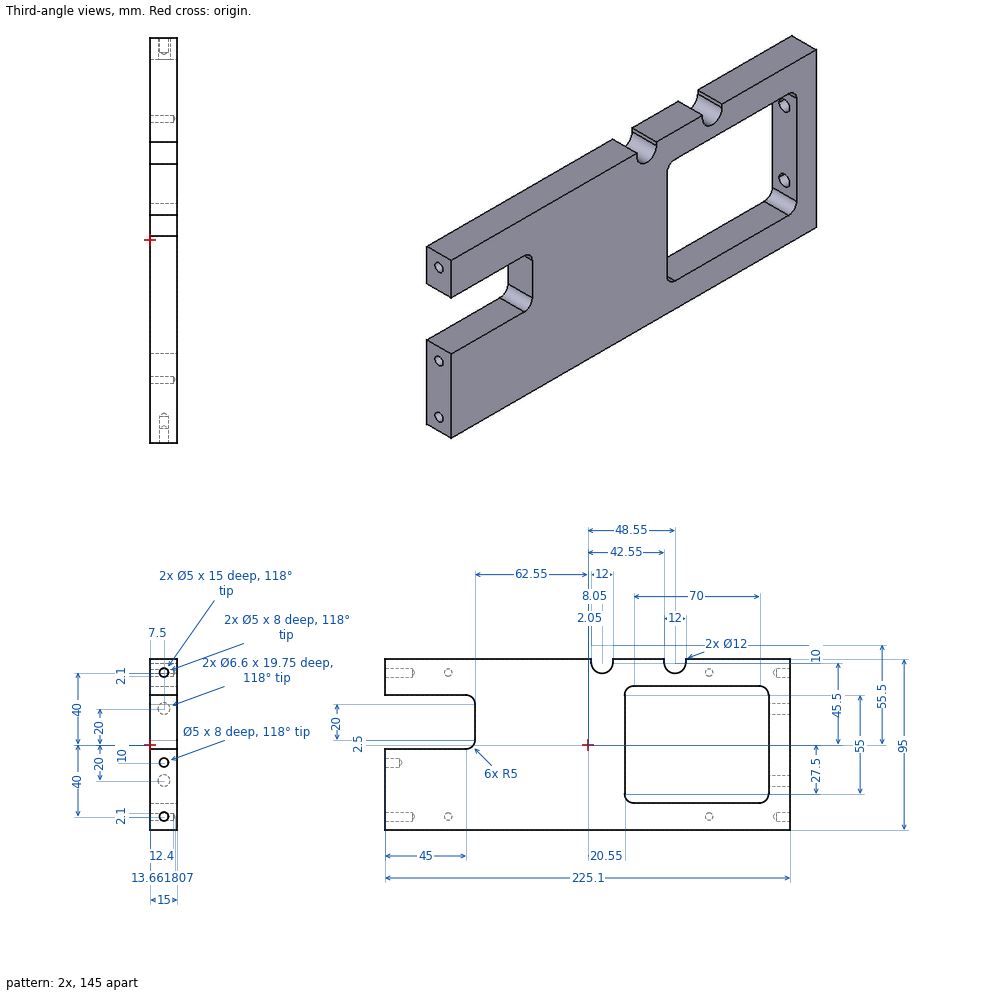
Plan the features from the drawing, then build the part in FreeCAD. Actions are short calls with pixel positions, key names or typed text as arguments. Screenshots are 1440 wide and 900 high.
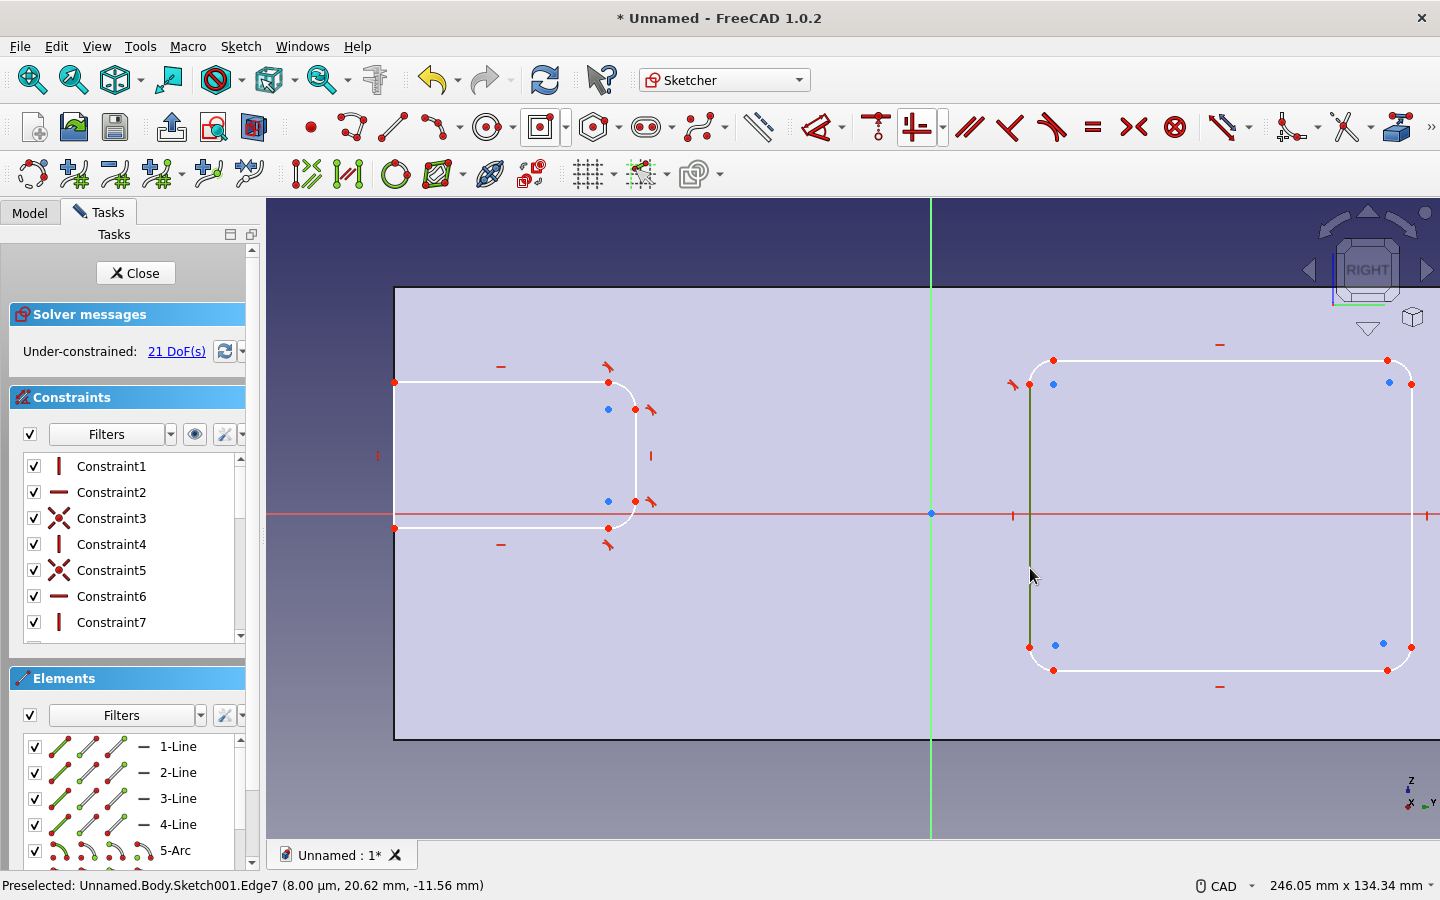
scroll(1033, 658, up, 2)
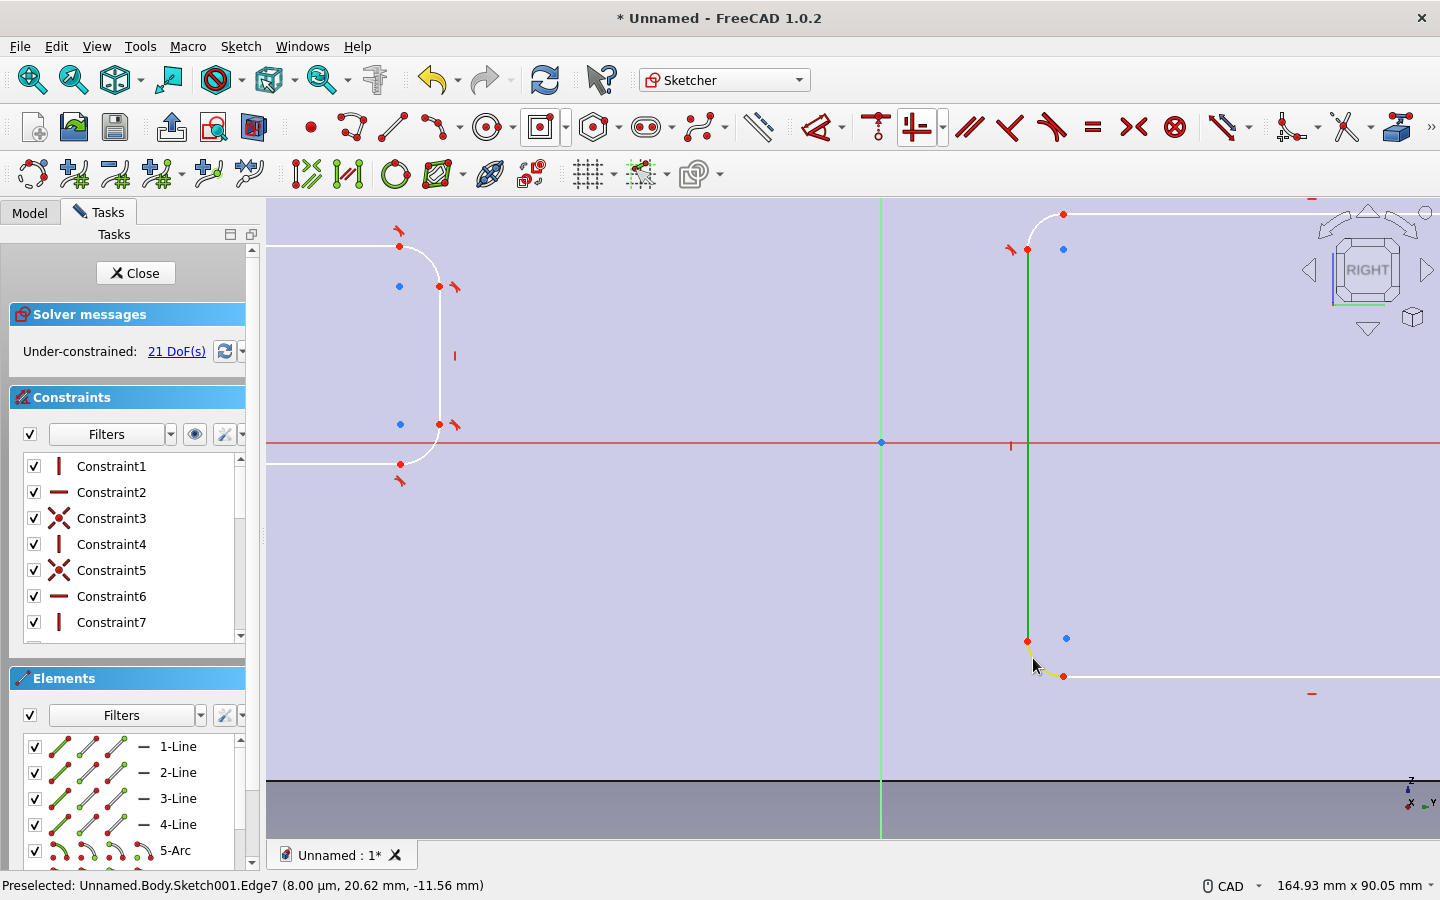
click(1032, 657)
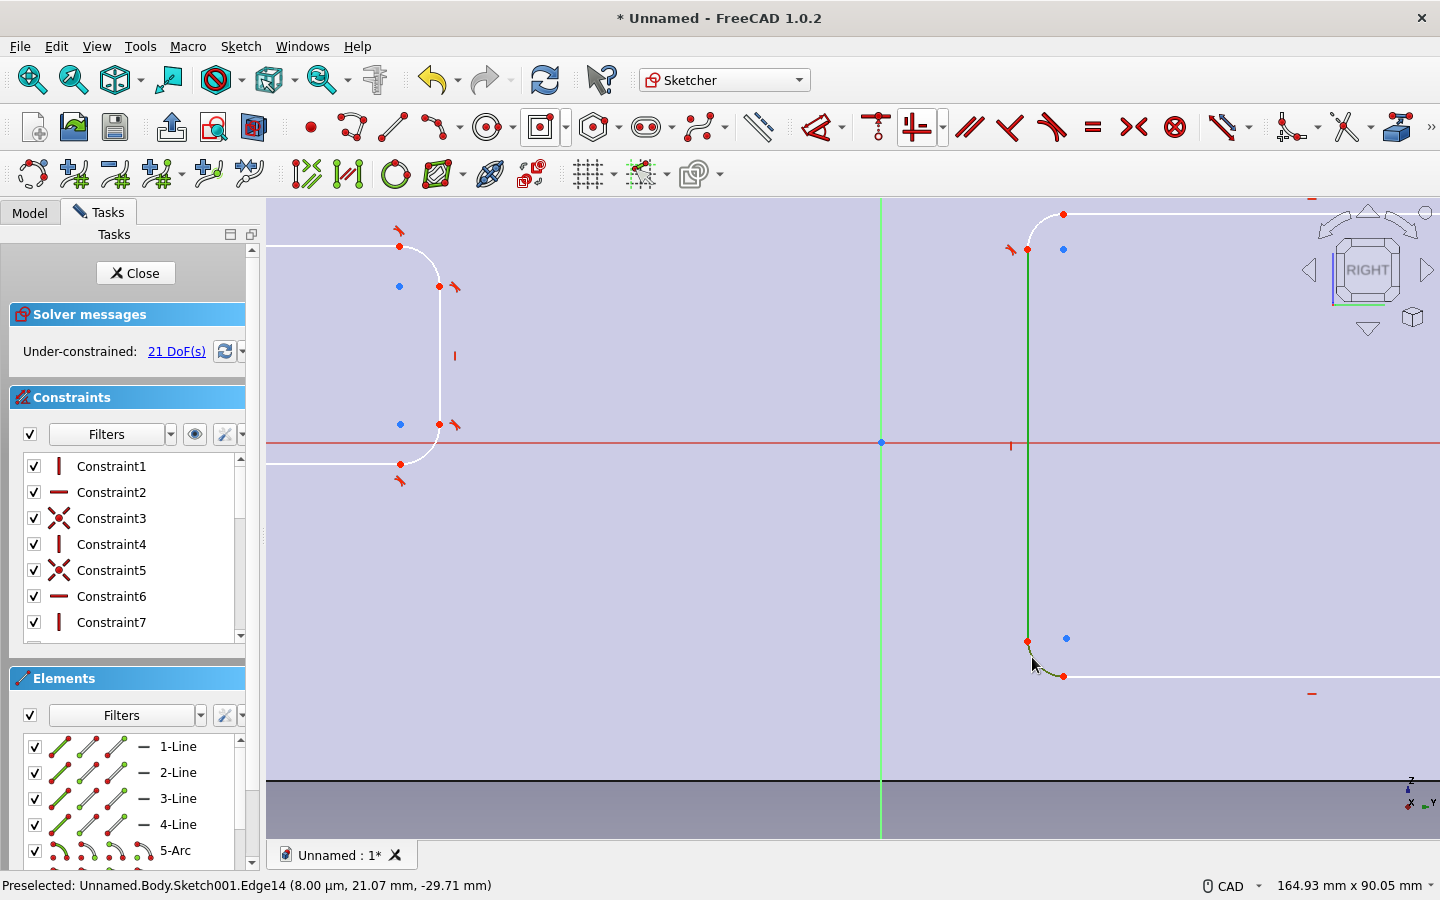
click(1052, 128)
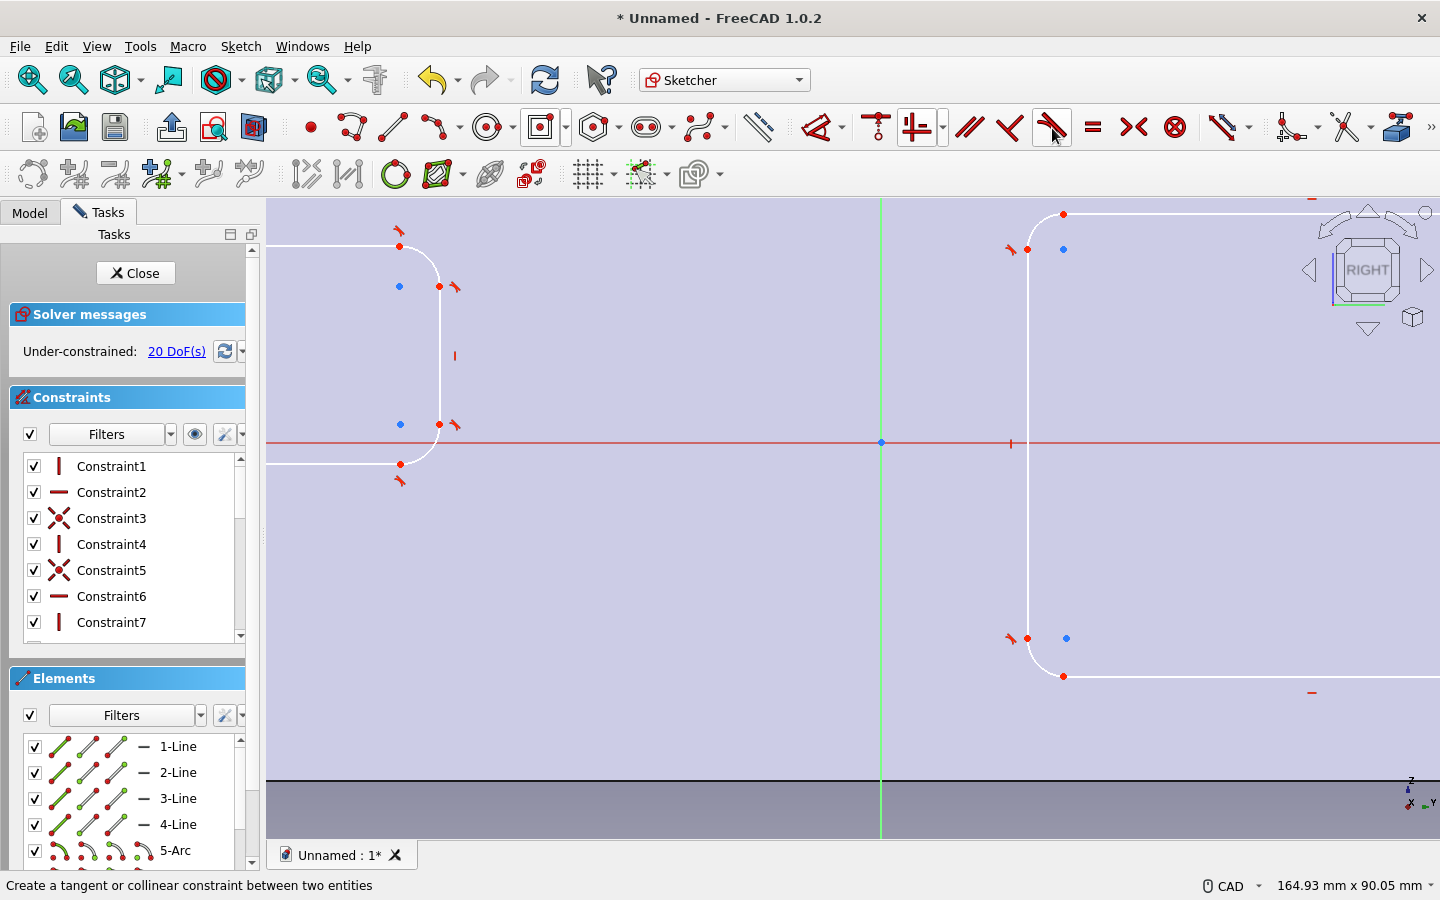
scroll(741, 580, down, 4)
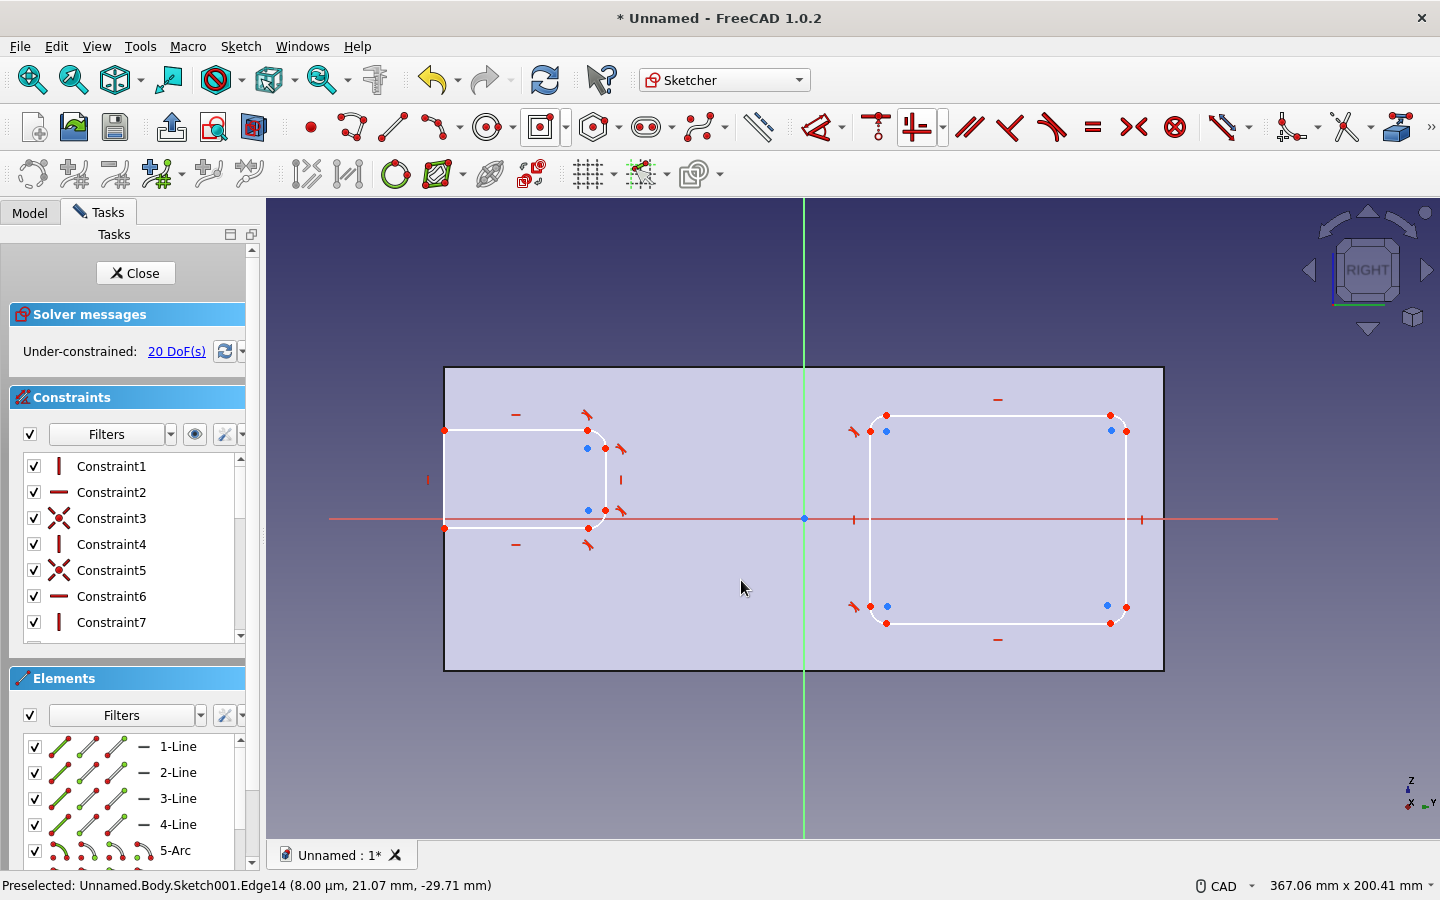
click(953, 416)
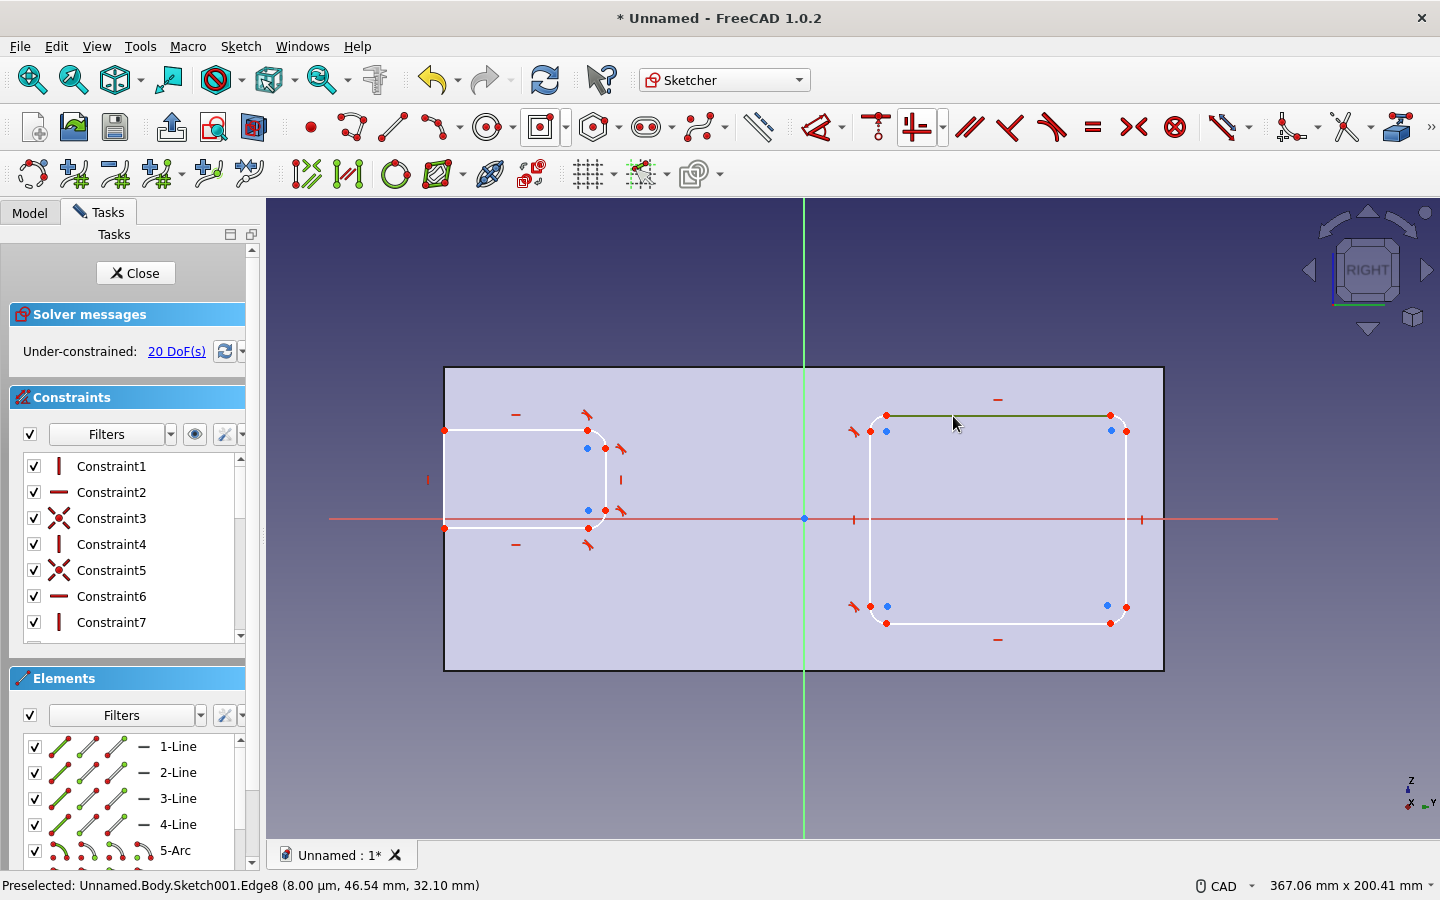
click(875, 421)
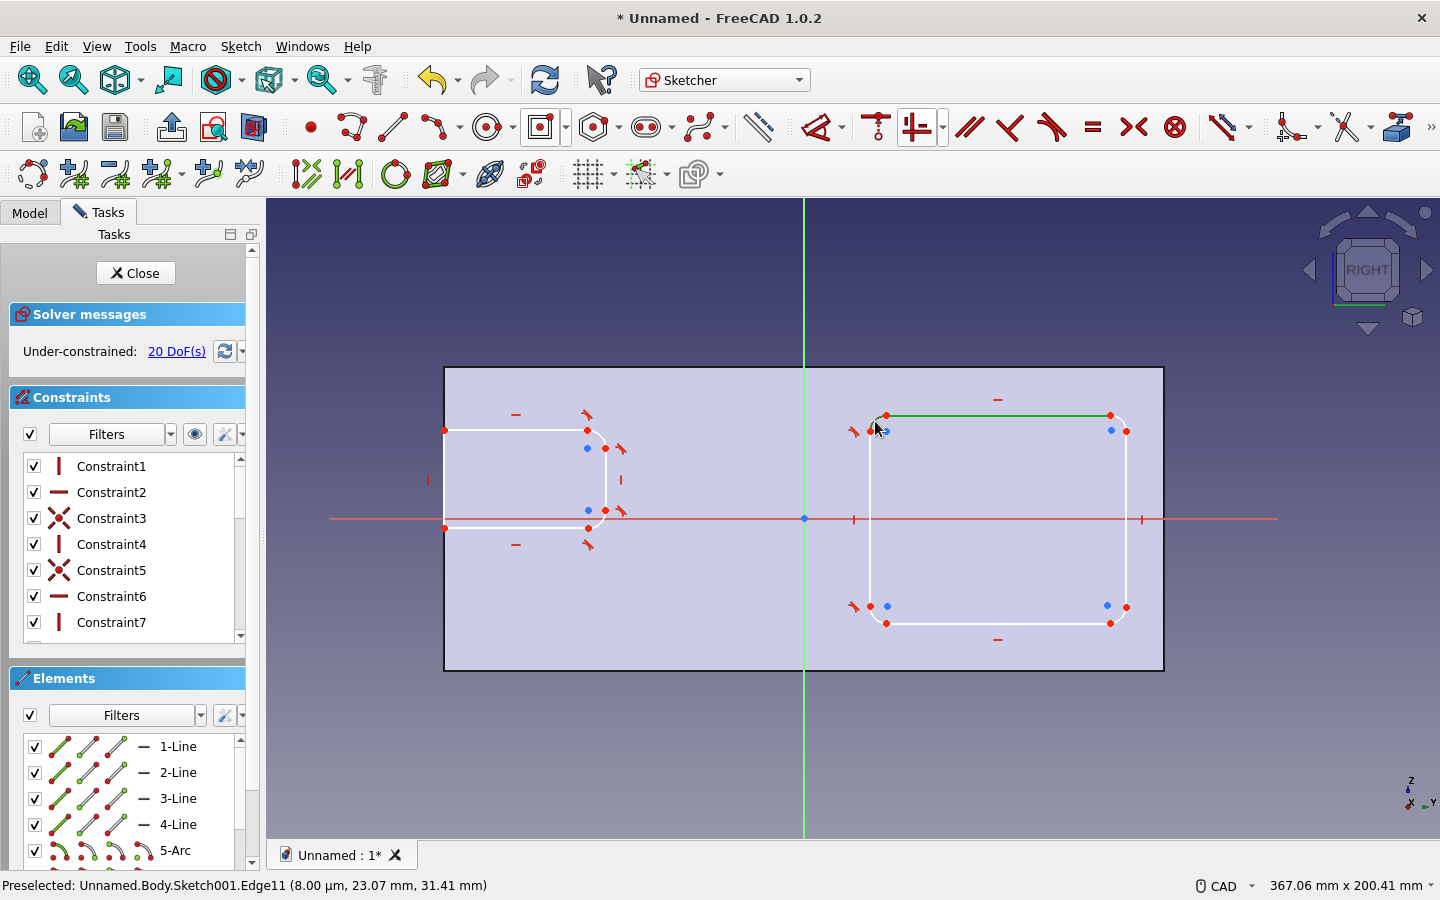
click(1052, 128)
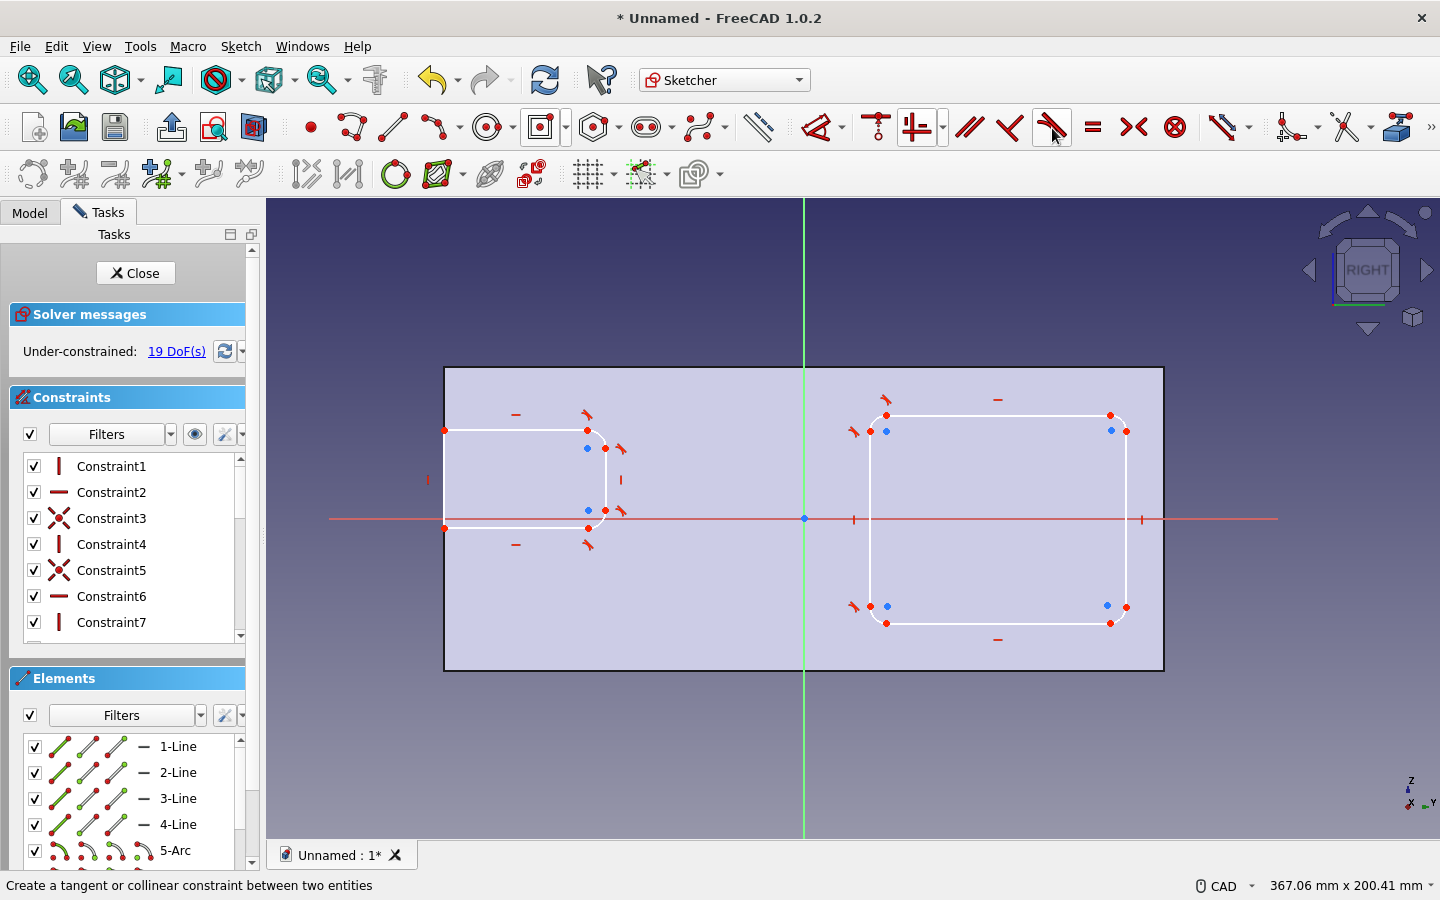
click(953, 416)